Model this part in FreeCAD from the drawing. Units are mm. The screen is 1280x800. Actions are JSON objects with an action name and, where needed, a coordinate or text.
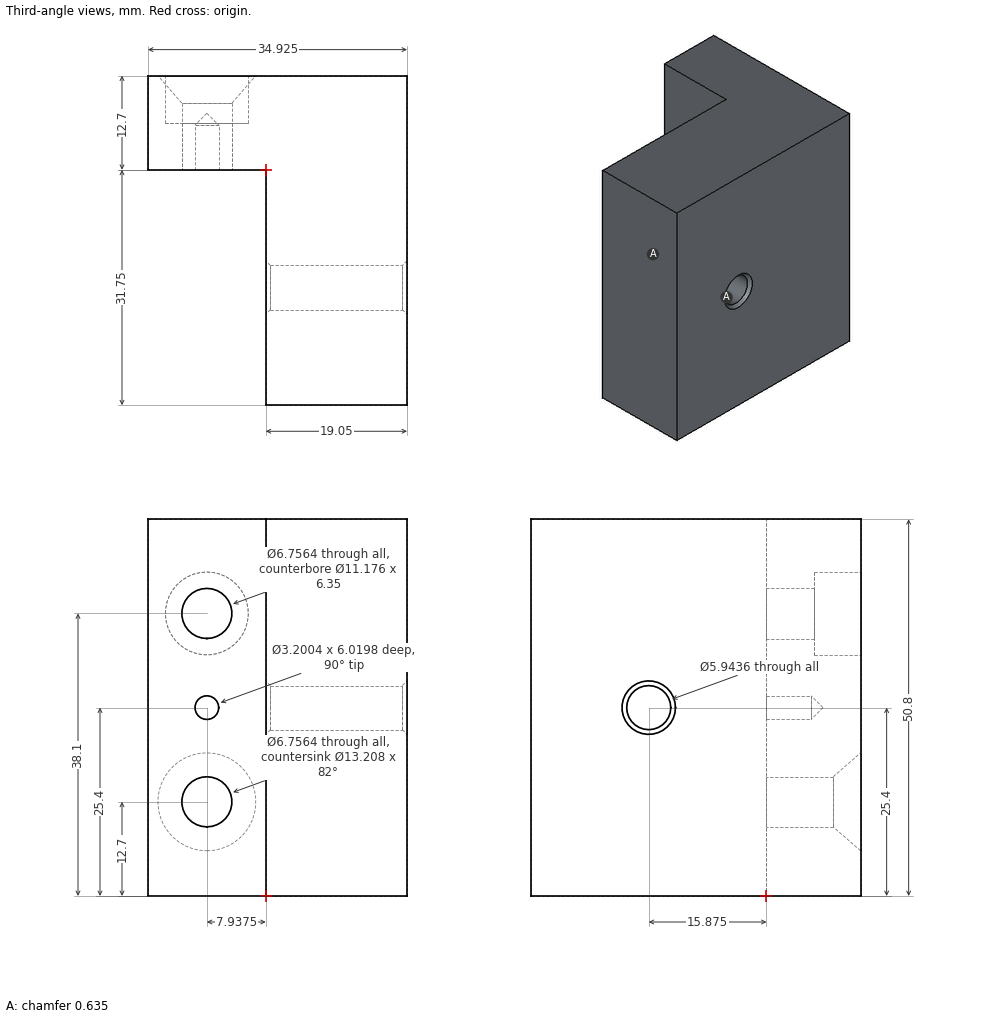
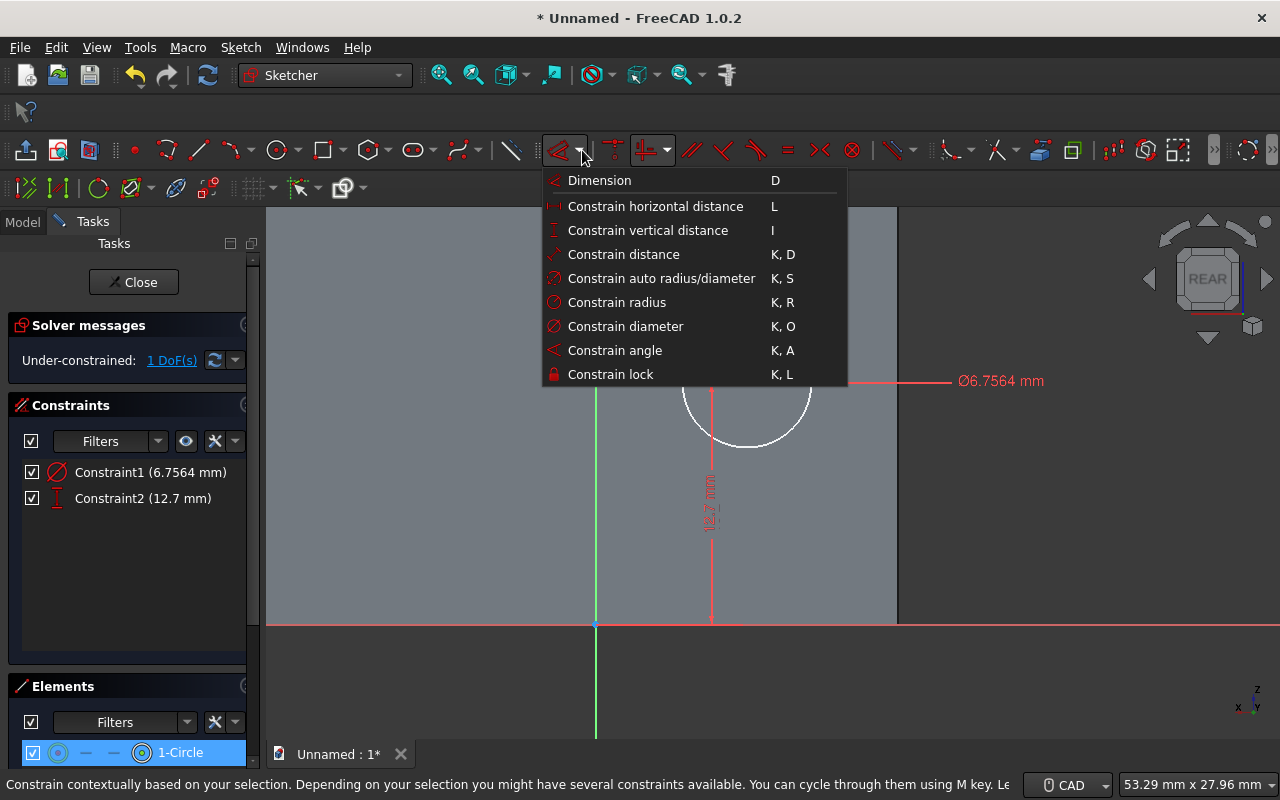
{"action": "left_click", "coordinate": [695, 206]}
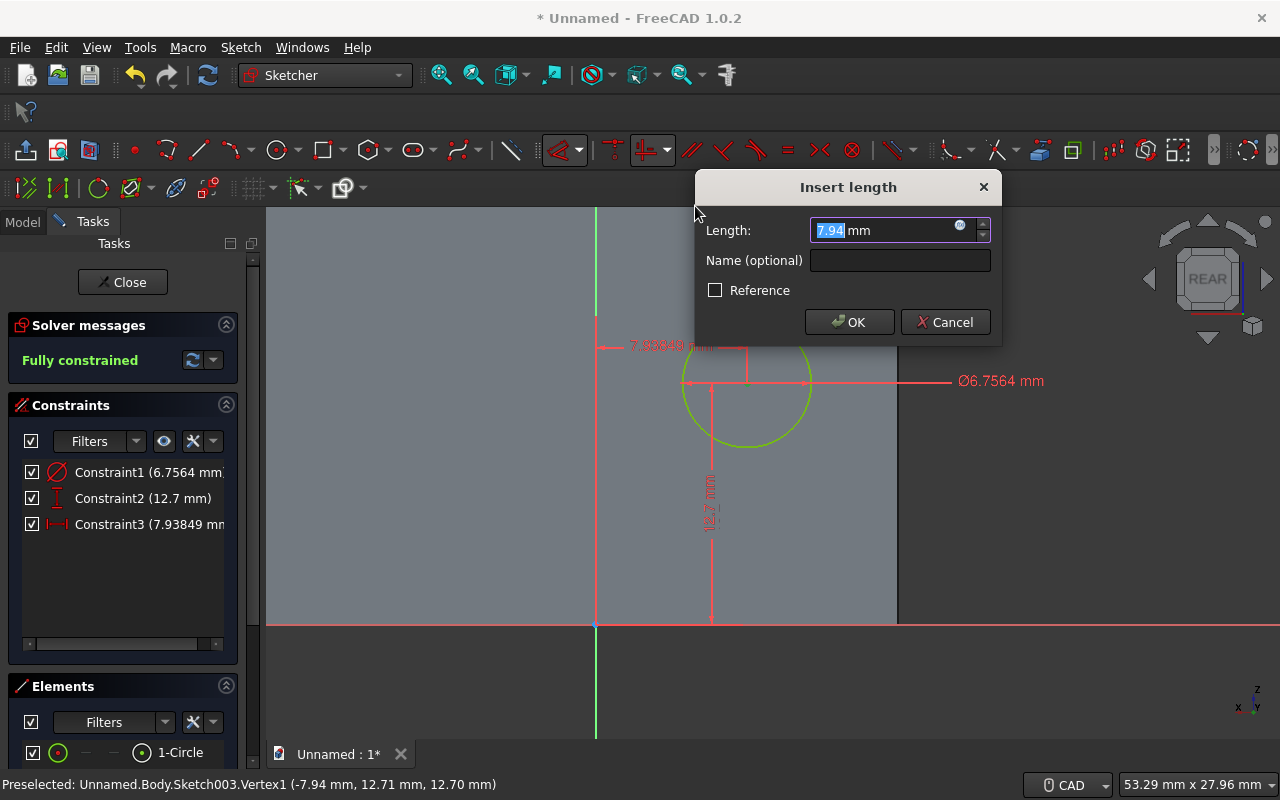
{"action": "type", "text": "7.9375"}
{"action": "key", "text": "Return"}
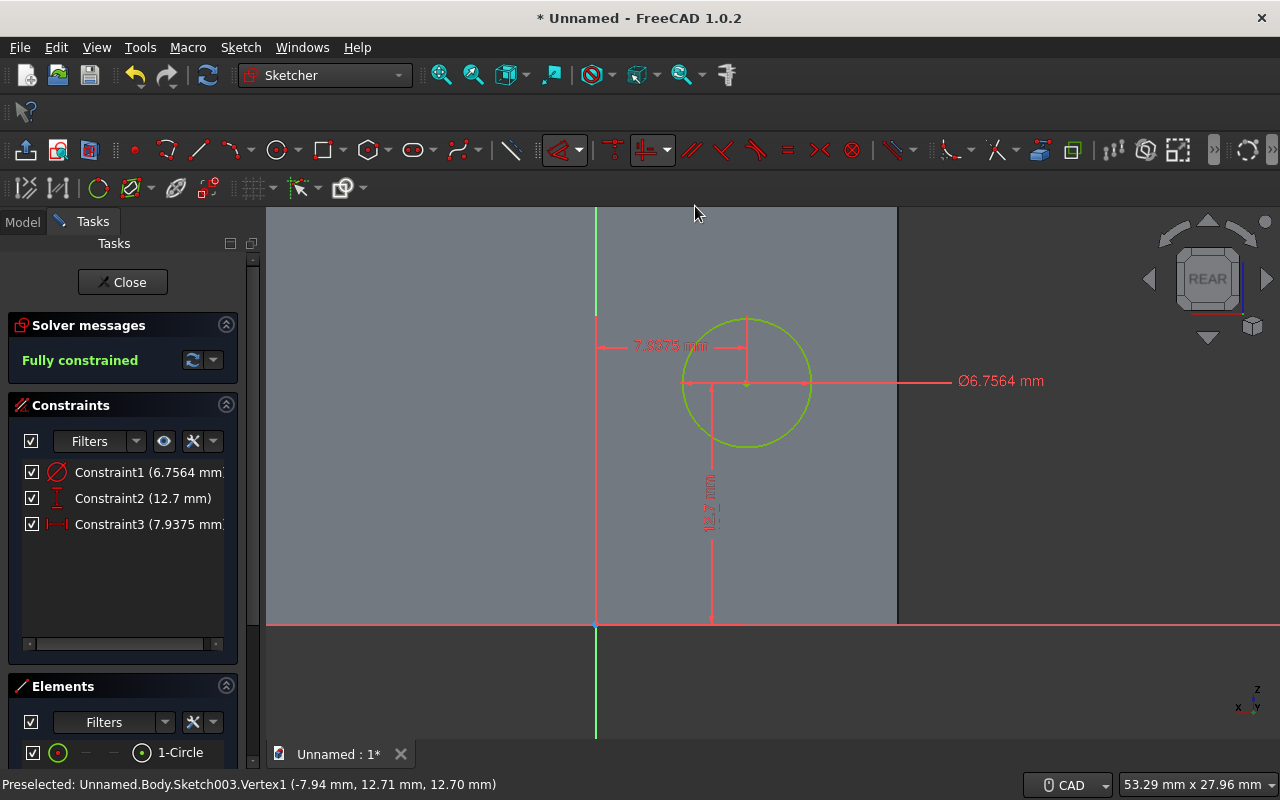
{"action": "left_click", "coordinate": [123, 282]}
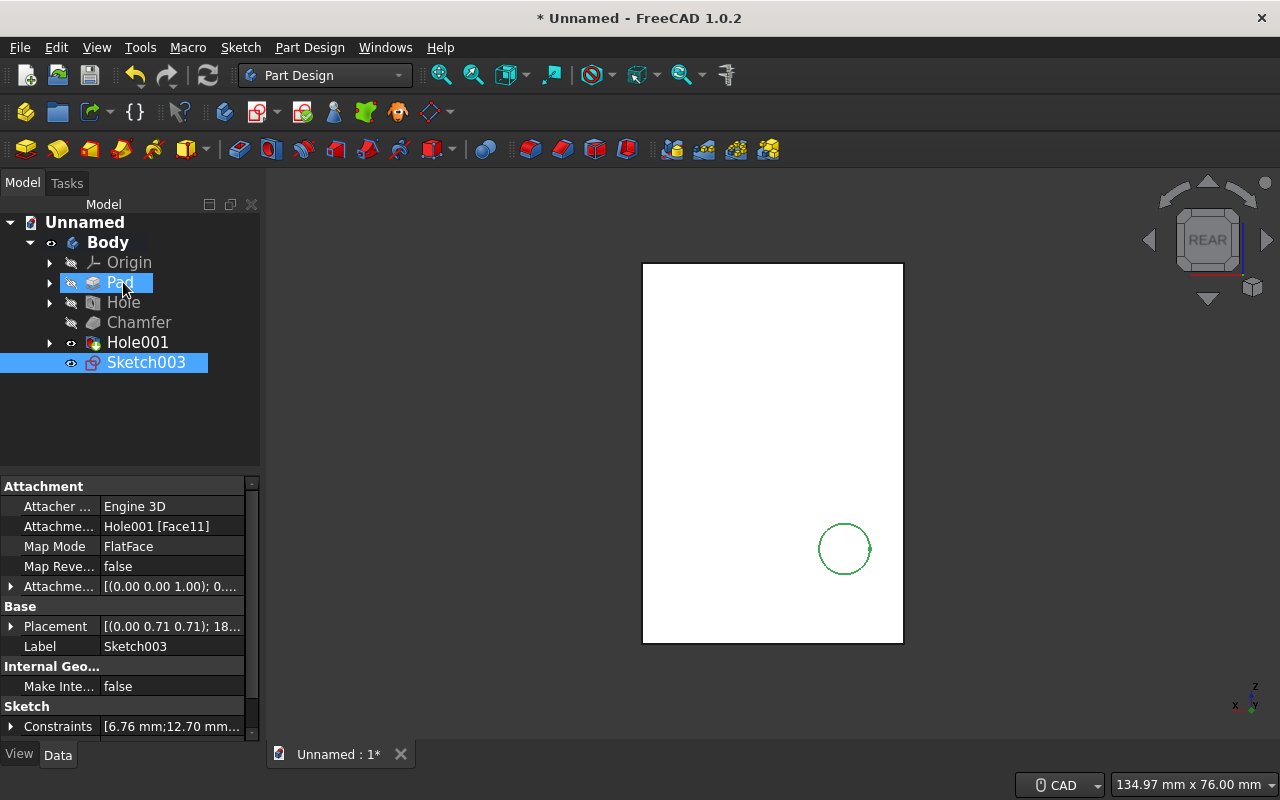
{"action": "left_click", "coordinate": [272, 150]}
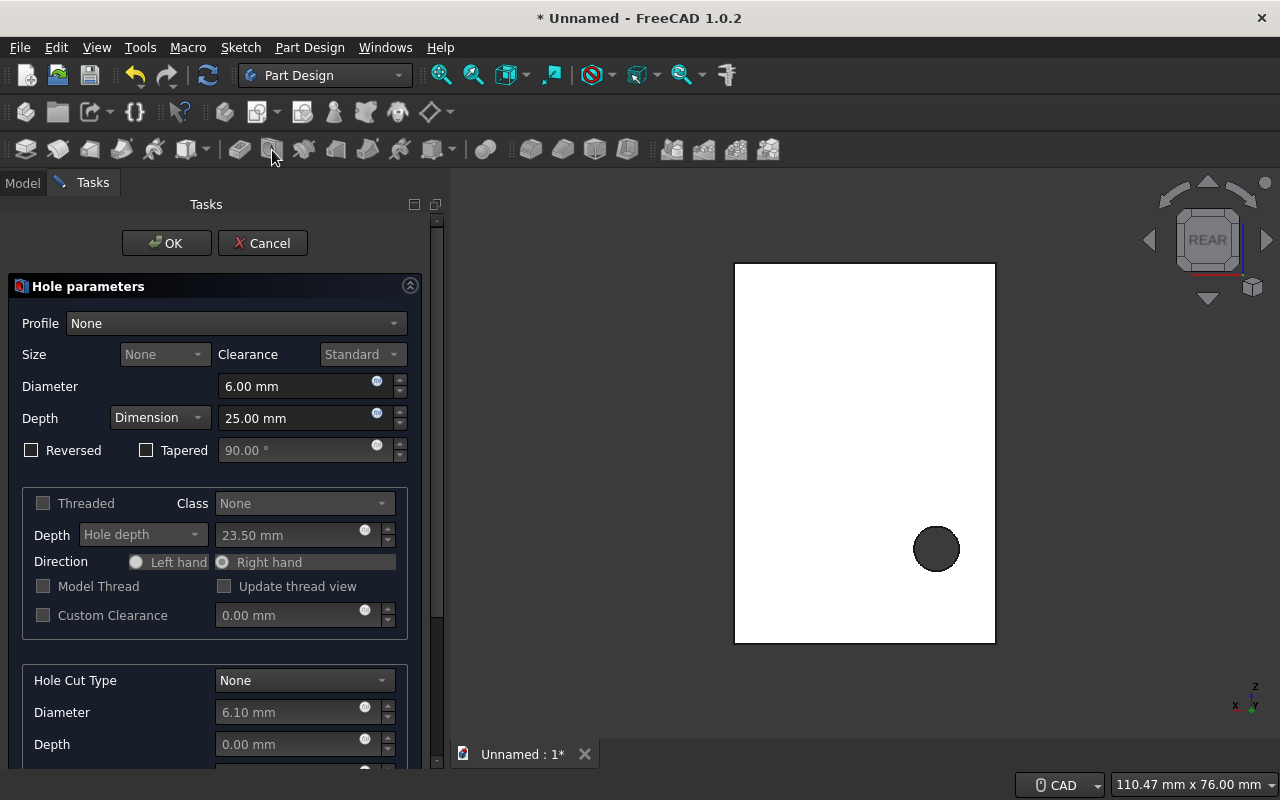
{"action": "triple_click", "coordinate": [305, 386]}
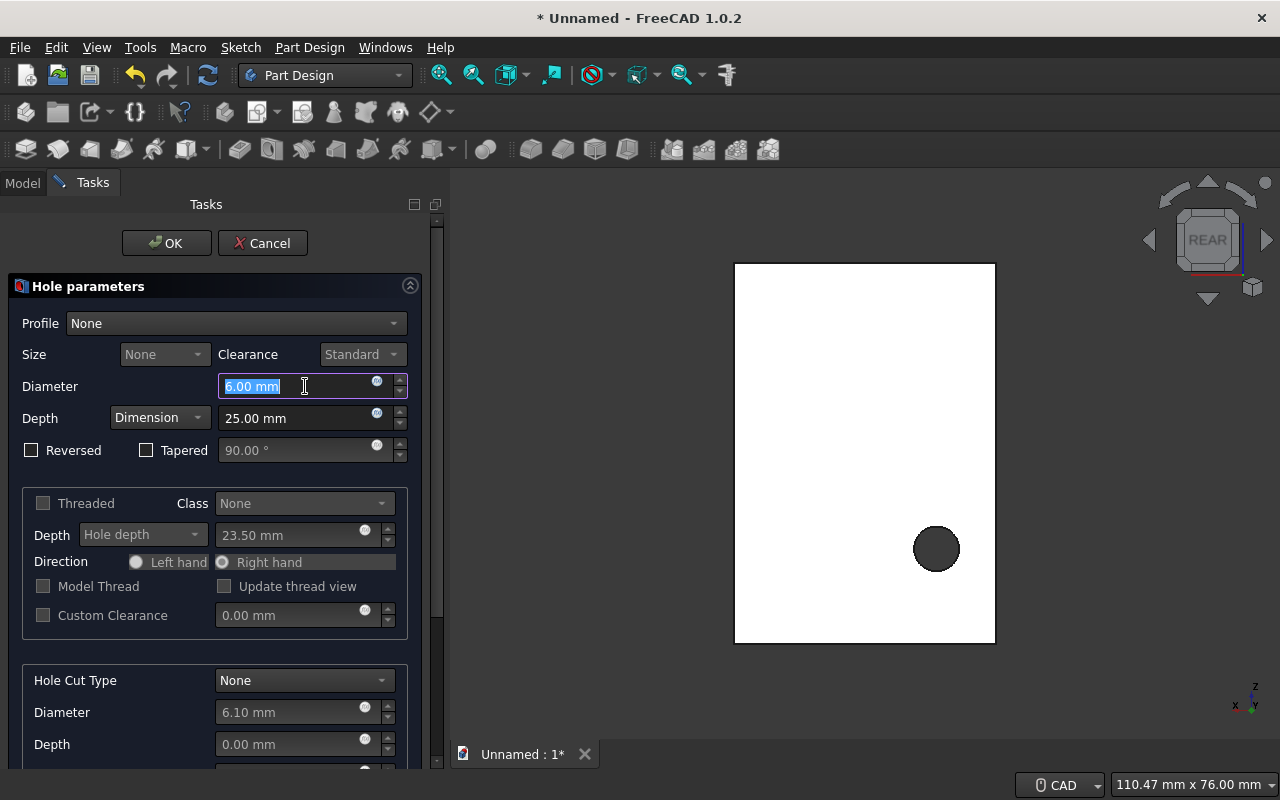
{"action": "type", "text": "6.7564"}
{"action": "key", "text": "Tab"}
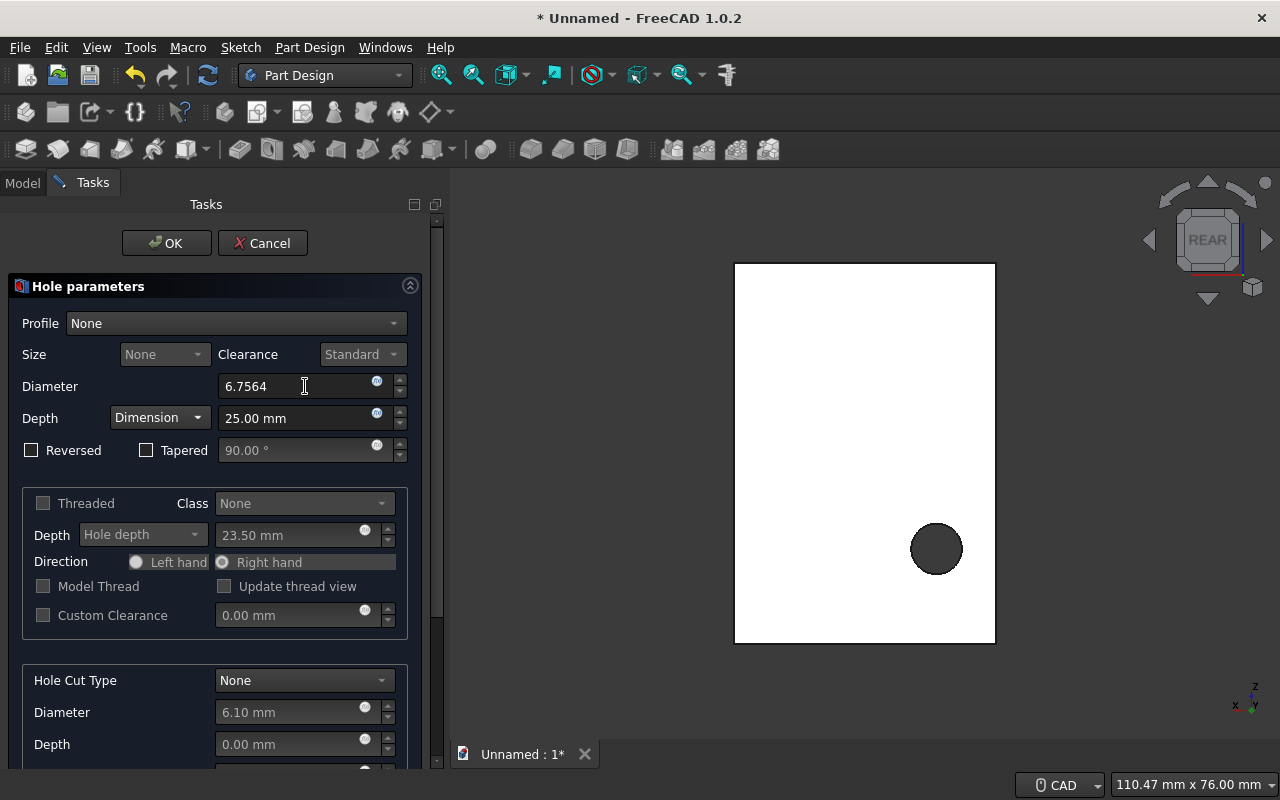
{"action": "left_click", "coordinate": [161, 418]}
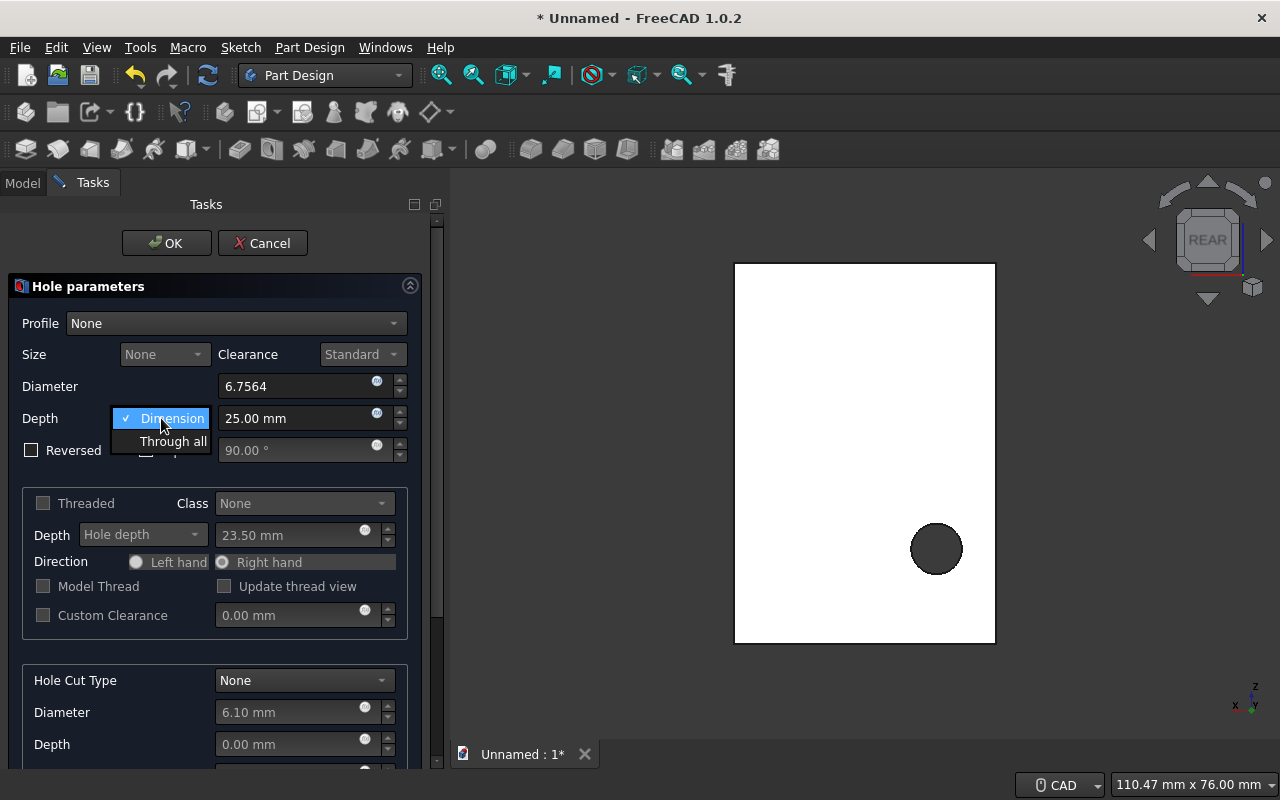
{"action": "left_click", "coordinate": [160, 442]}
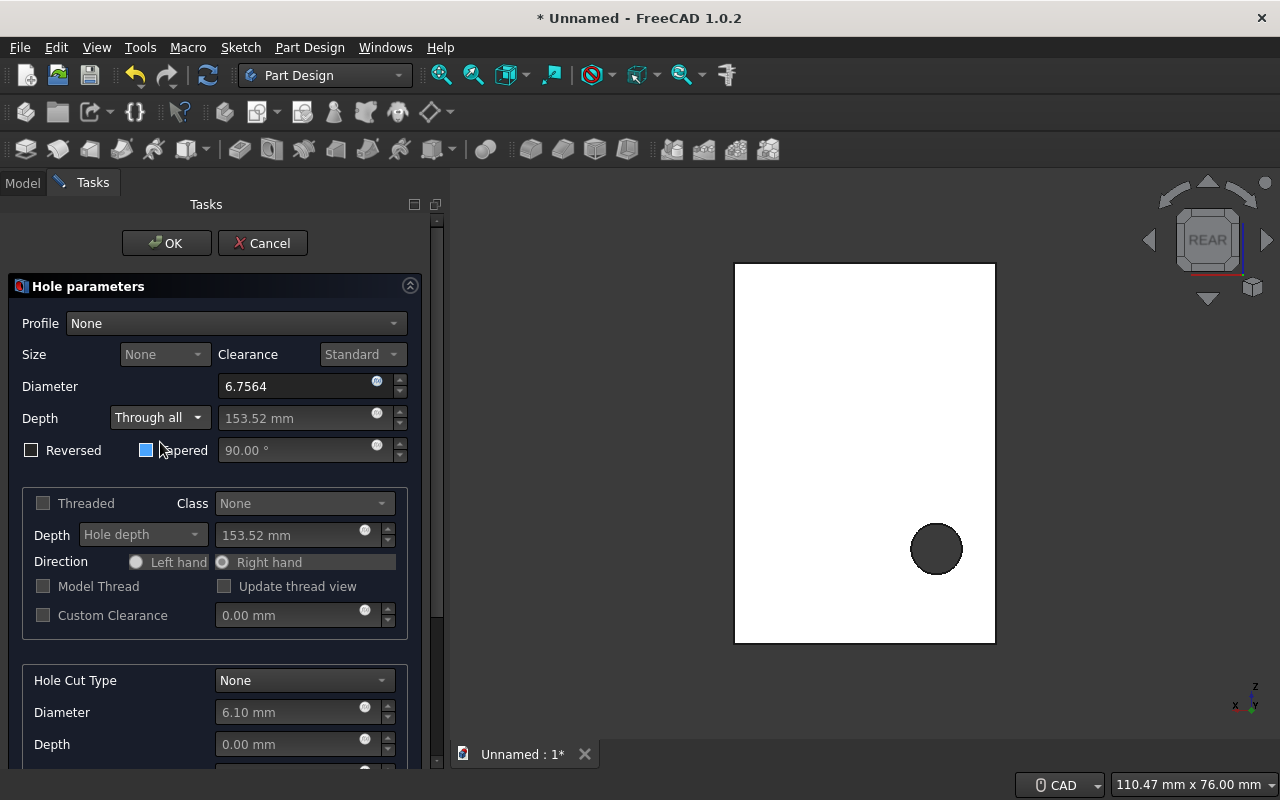
{"action": "left_click", "coordinate": [306, 680]}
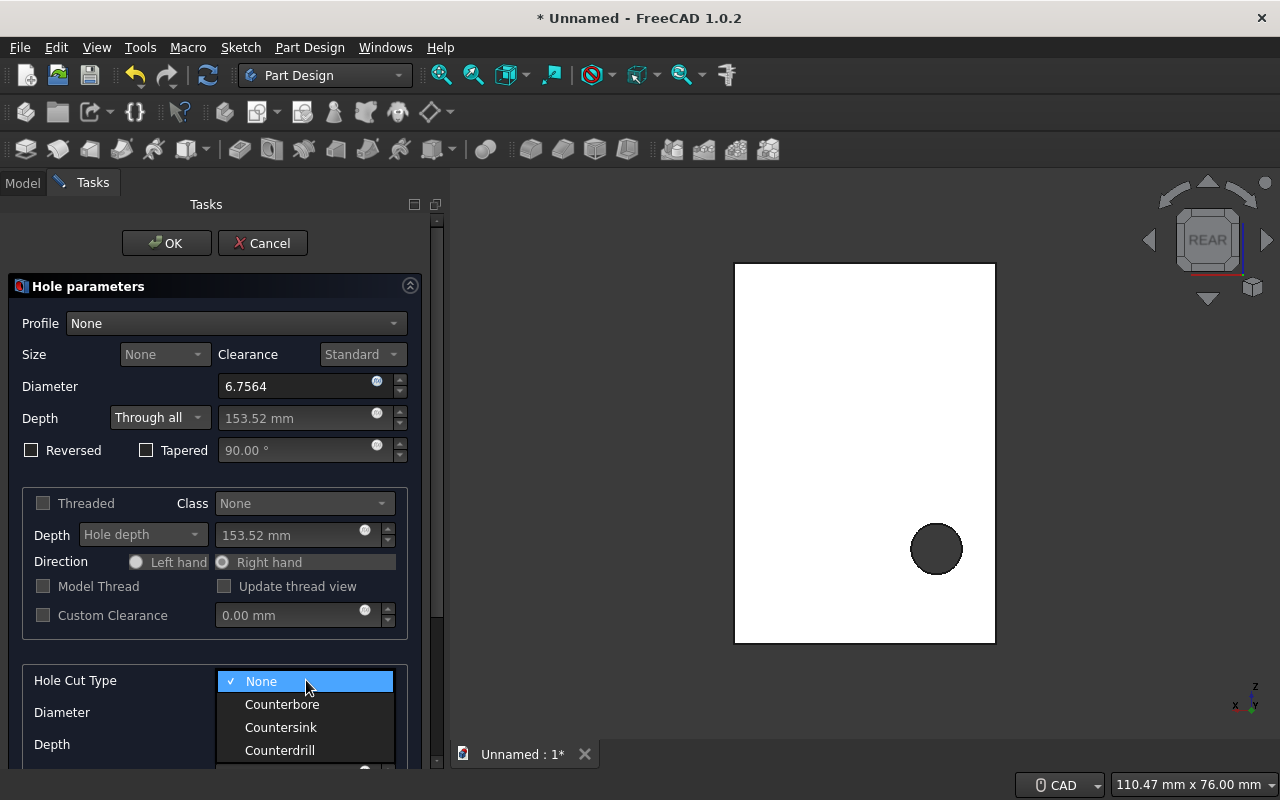
{"action": "left_click", "coordinate": [304, 728]}